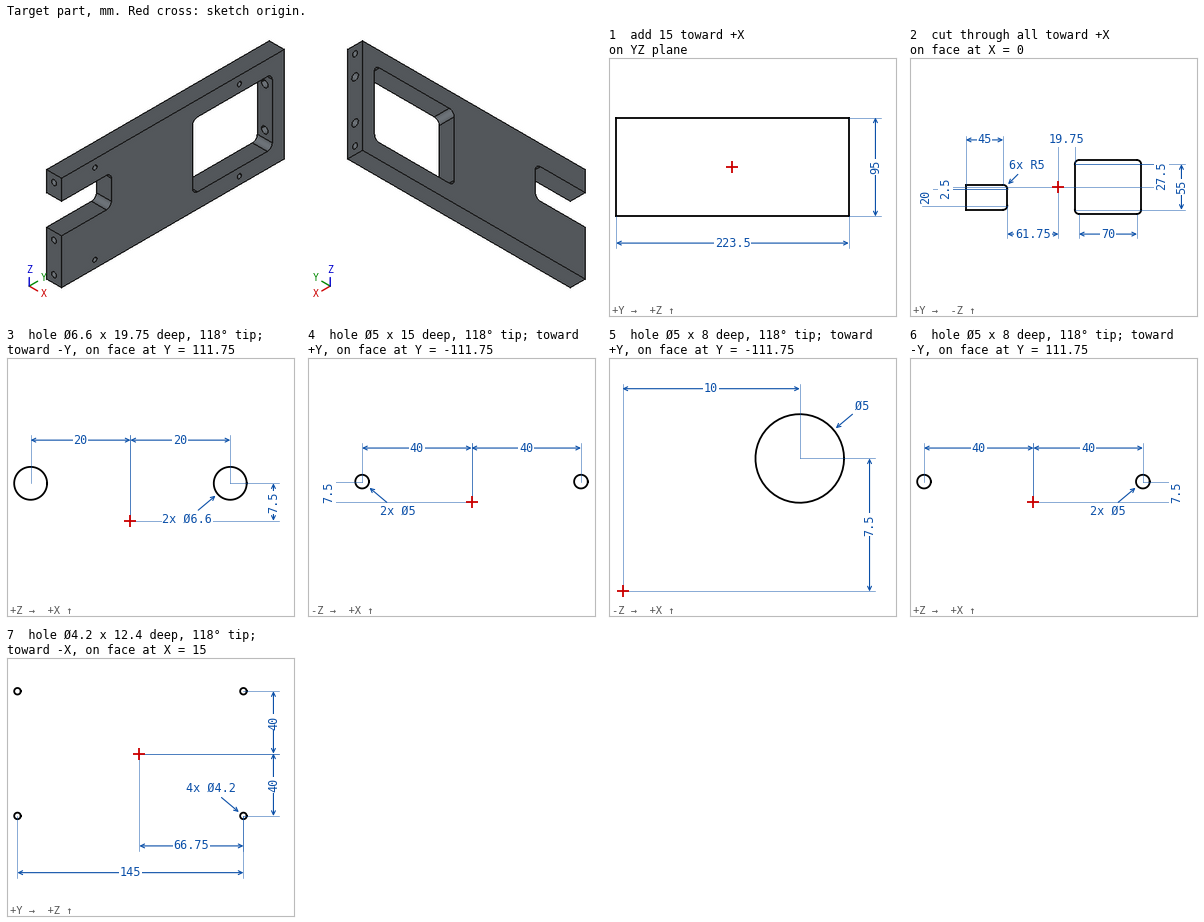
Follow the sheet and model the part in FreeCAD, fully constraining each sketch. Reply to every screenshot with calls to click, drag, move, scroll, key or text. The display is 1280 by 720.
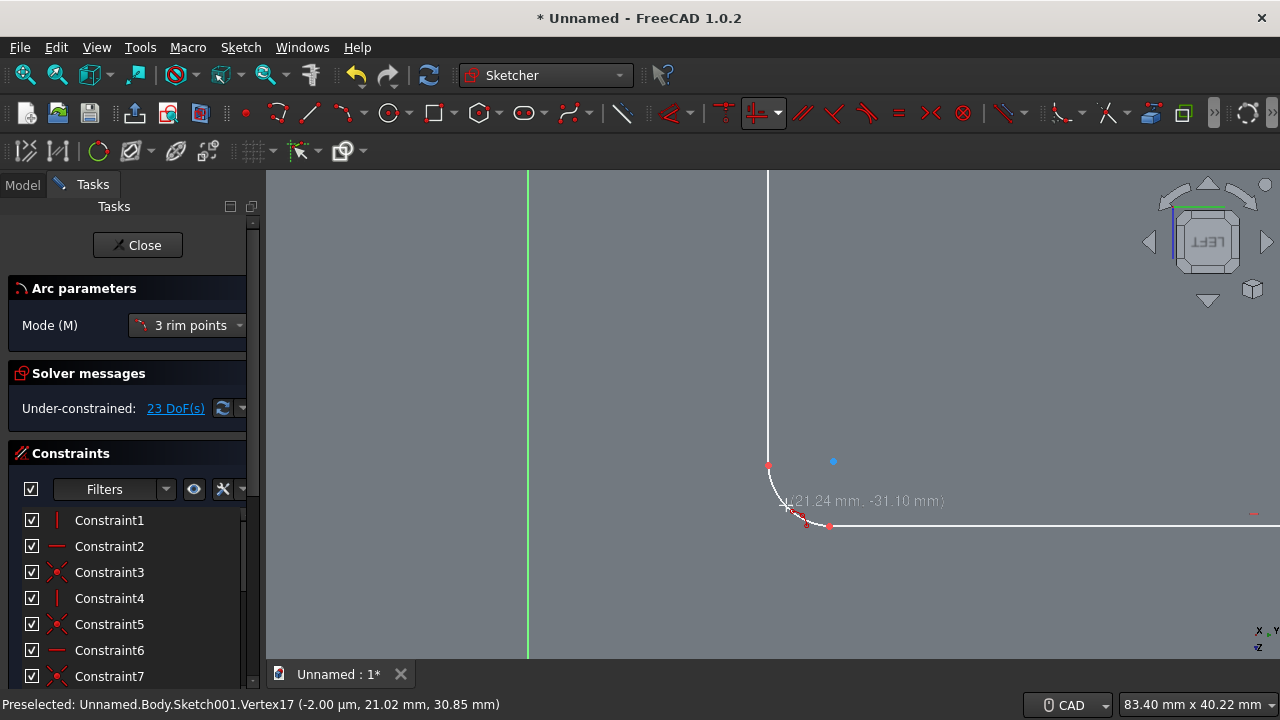
scroll(786, 508, down, 7)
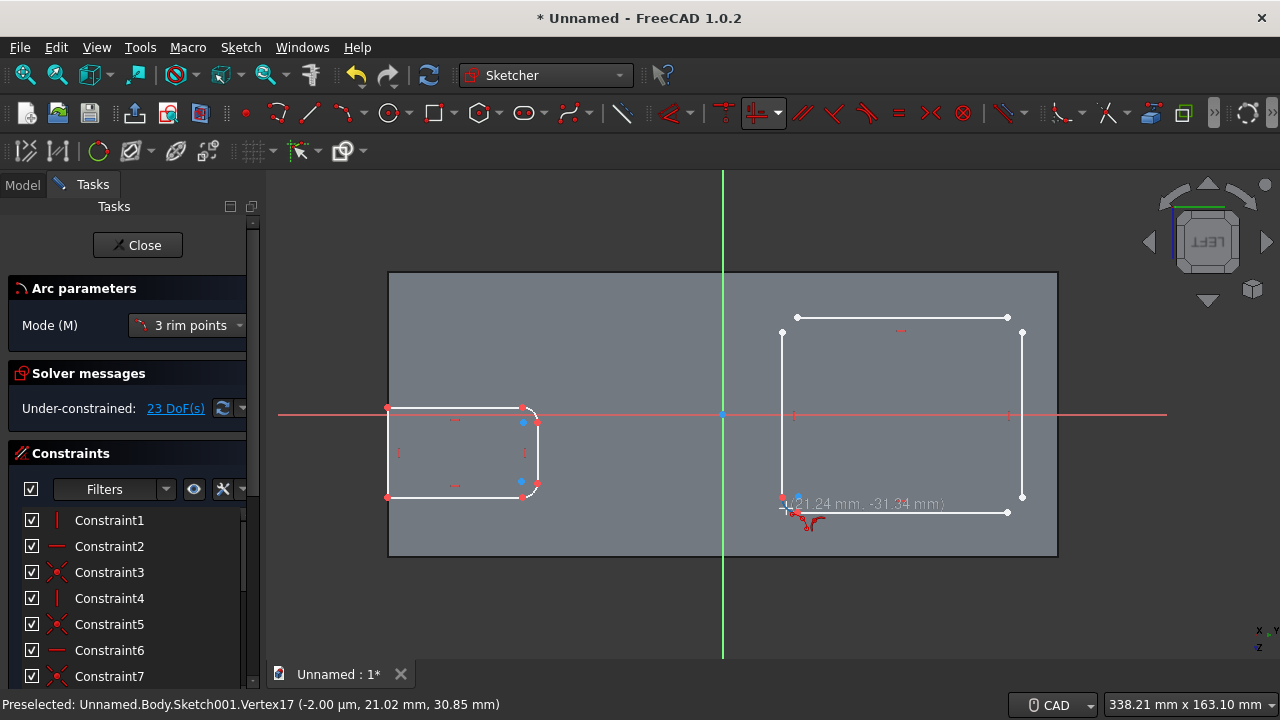
click(1007, 513)
click(1022, 498)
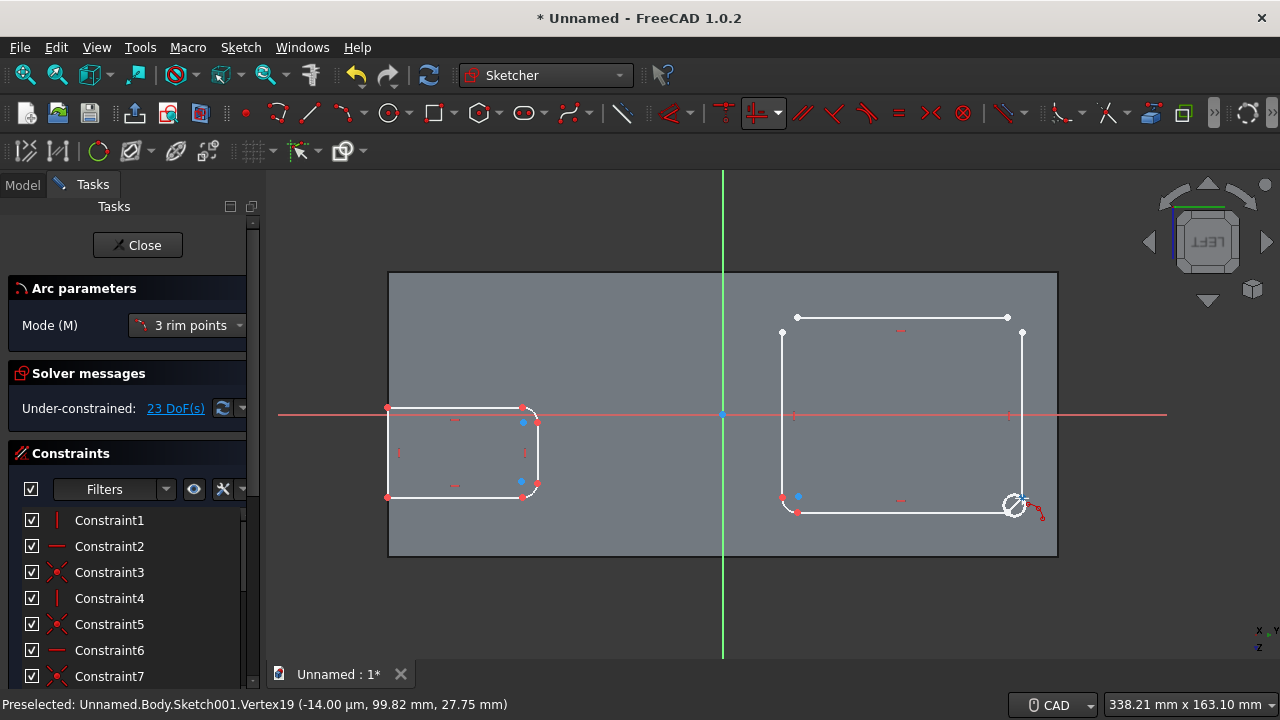
scroll(1017, 508, up, 7)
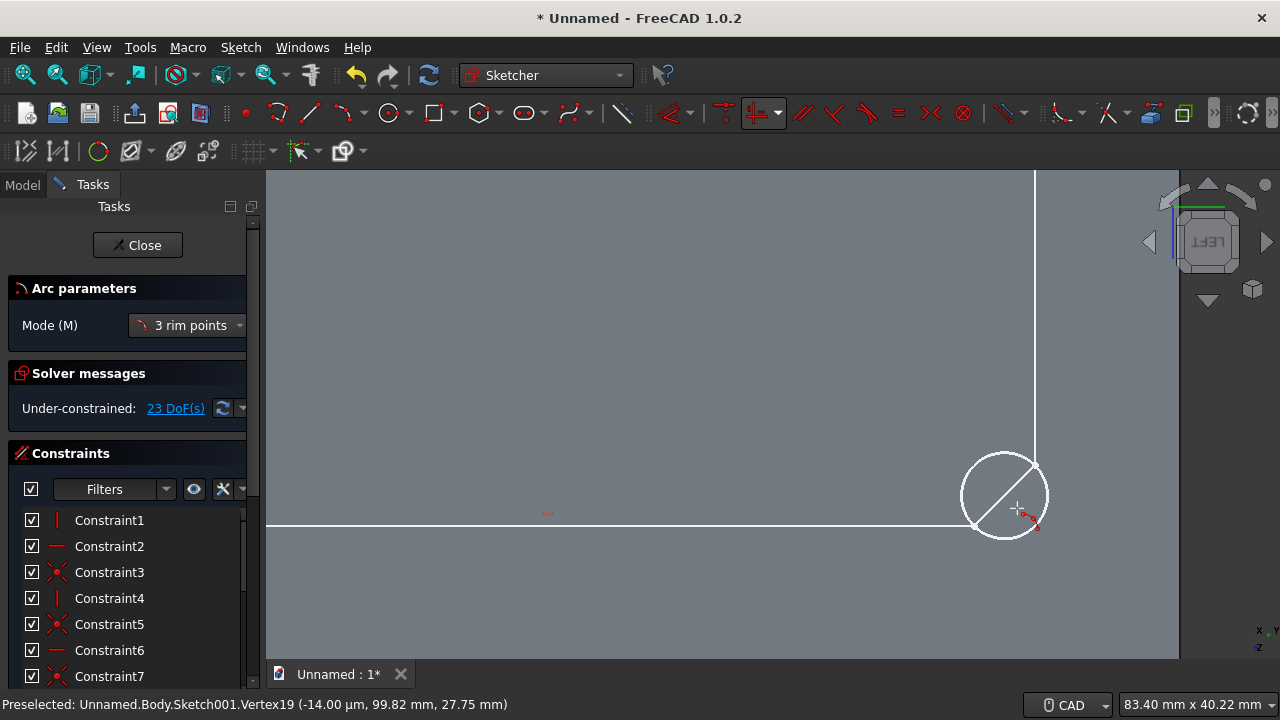
click(1016, 505)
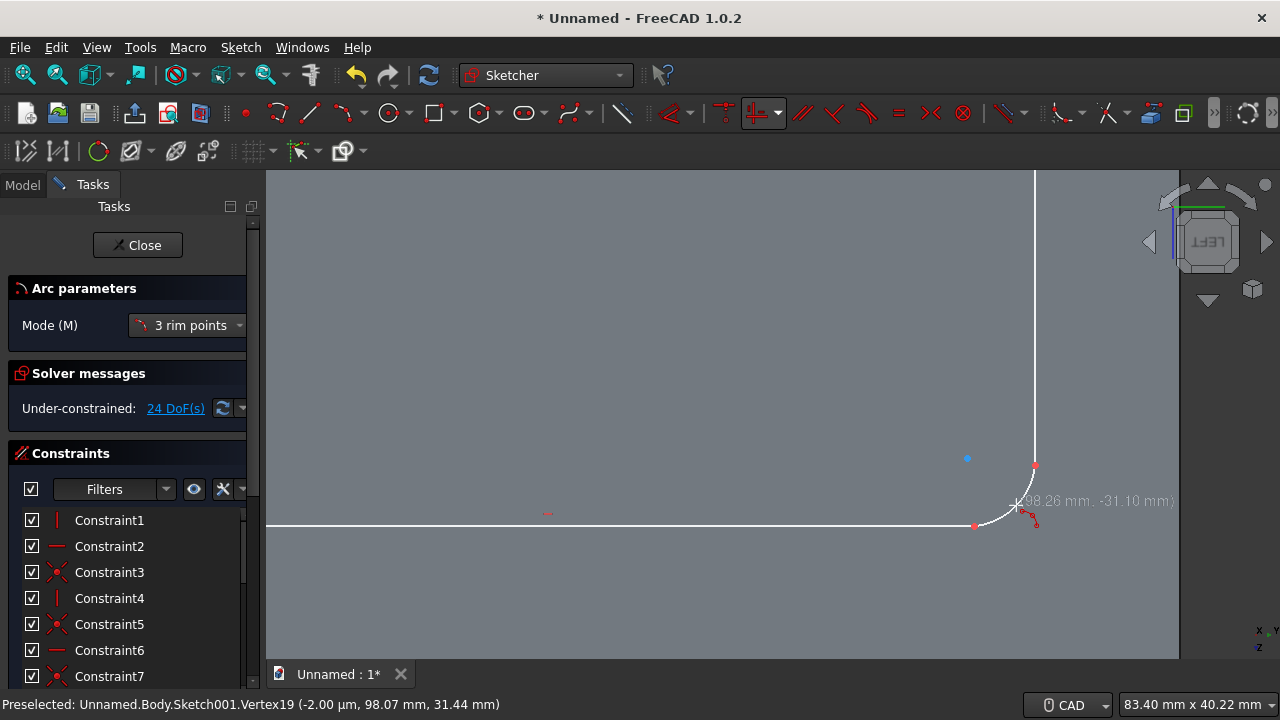
scroll(1017, 508, down, 7)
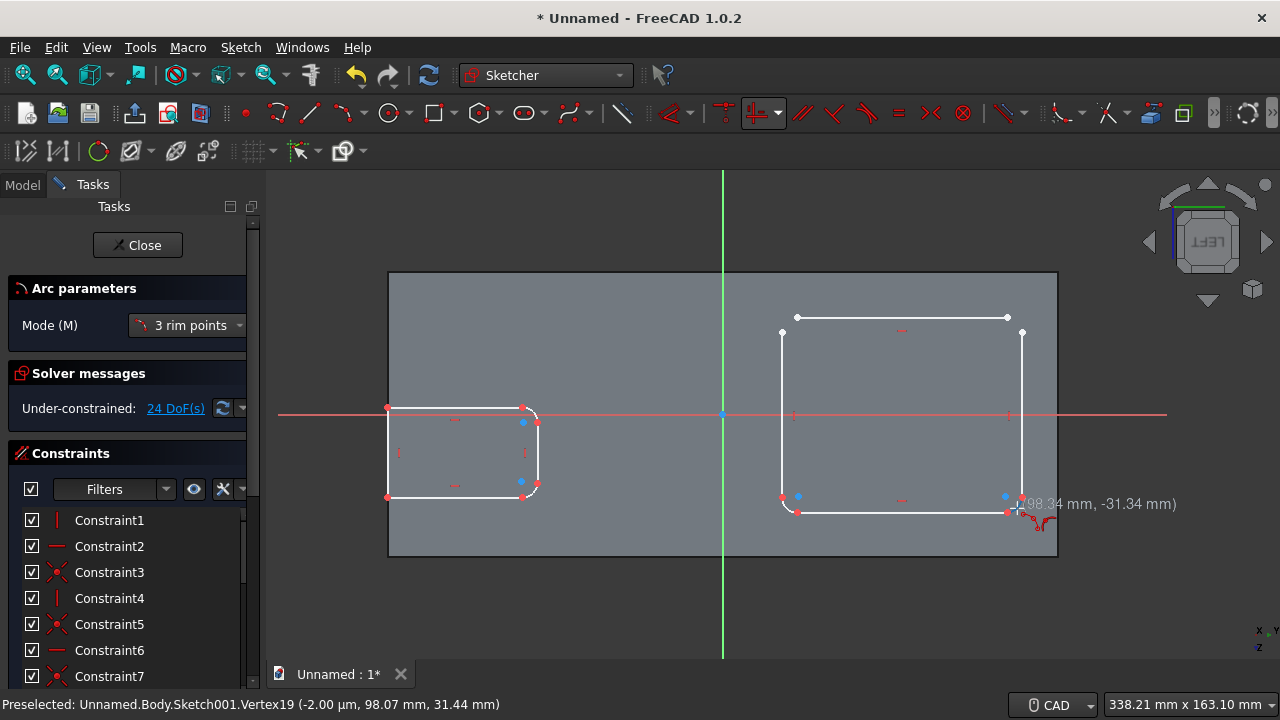
click(1022, 333)
click(1007, 318)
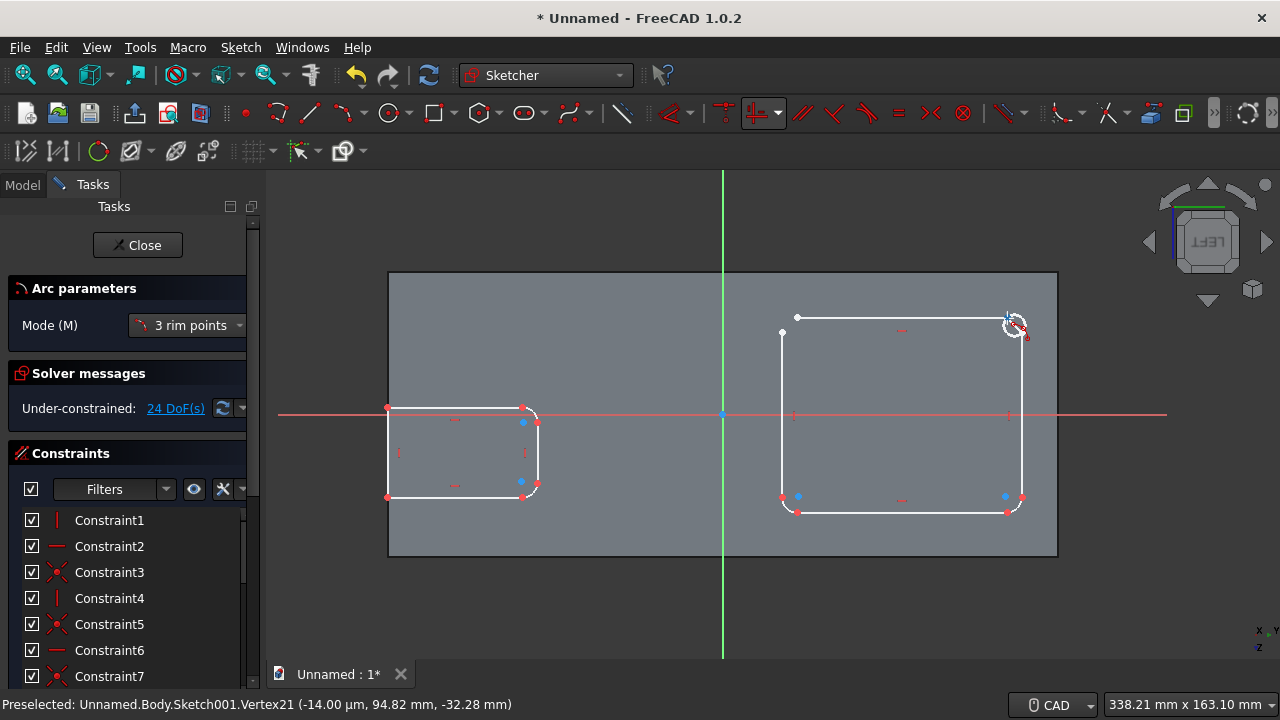
scroll(1017, 322, up, 7)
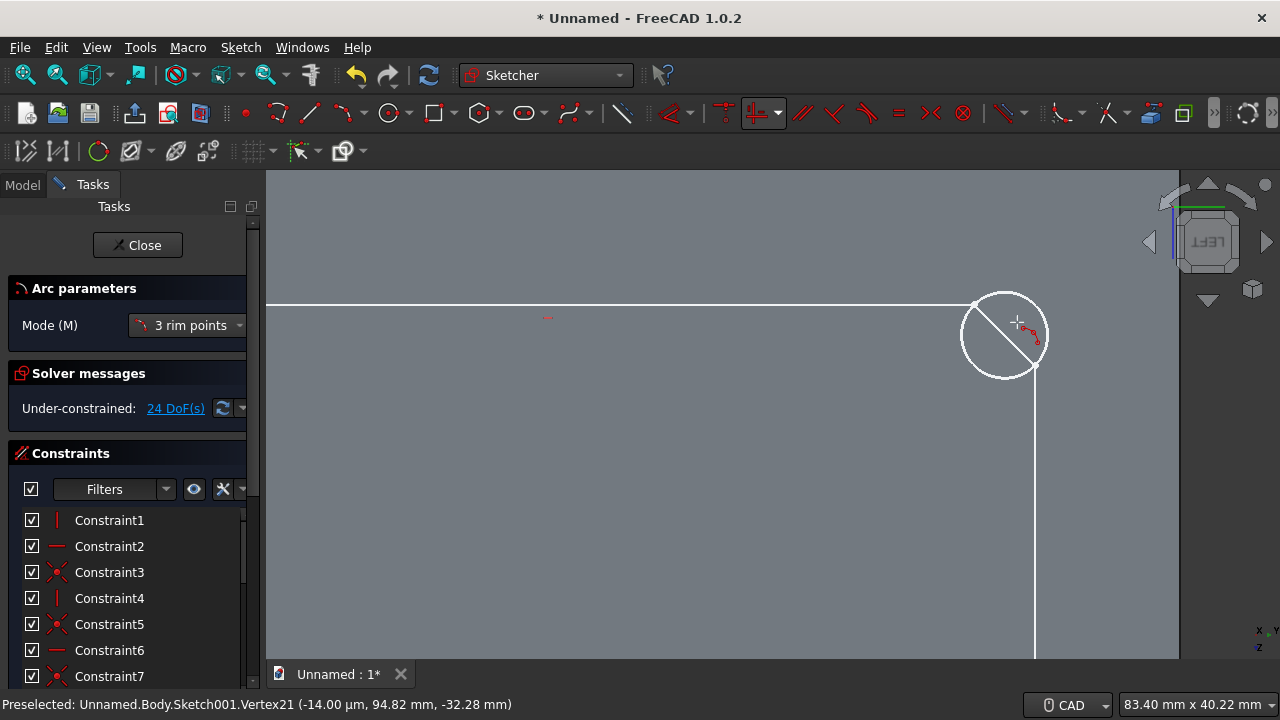
click(1016, 320)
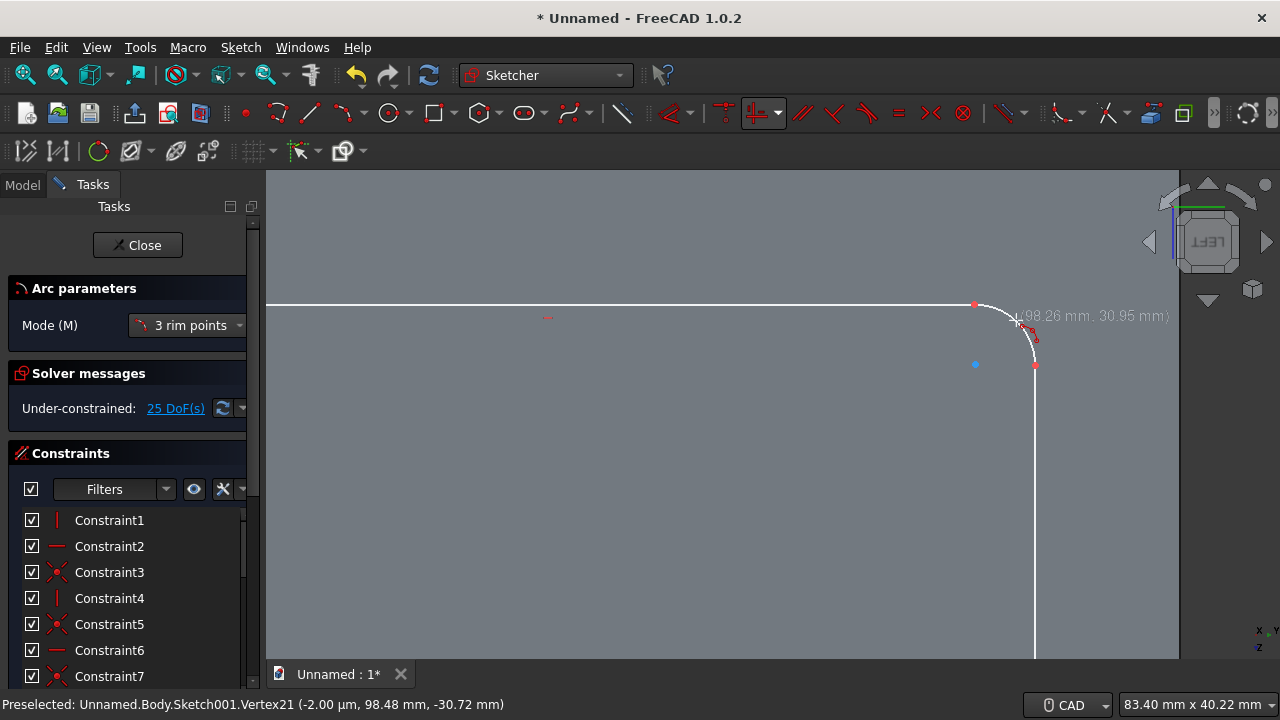
scroll(1017, 322, down, 7)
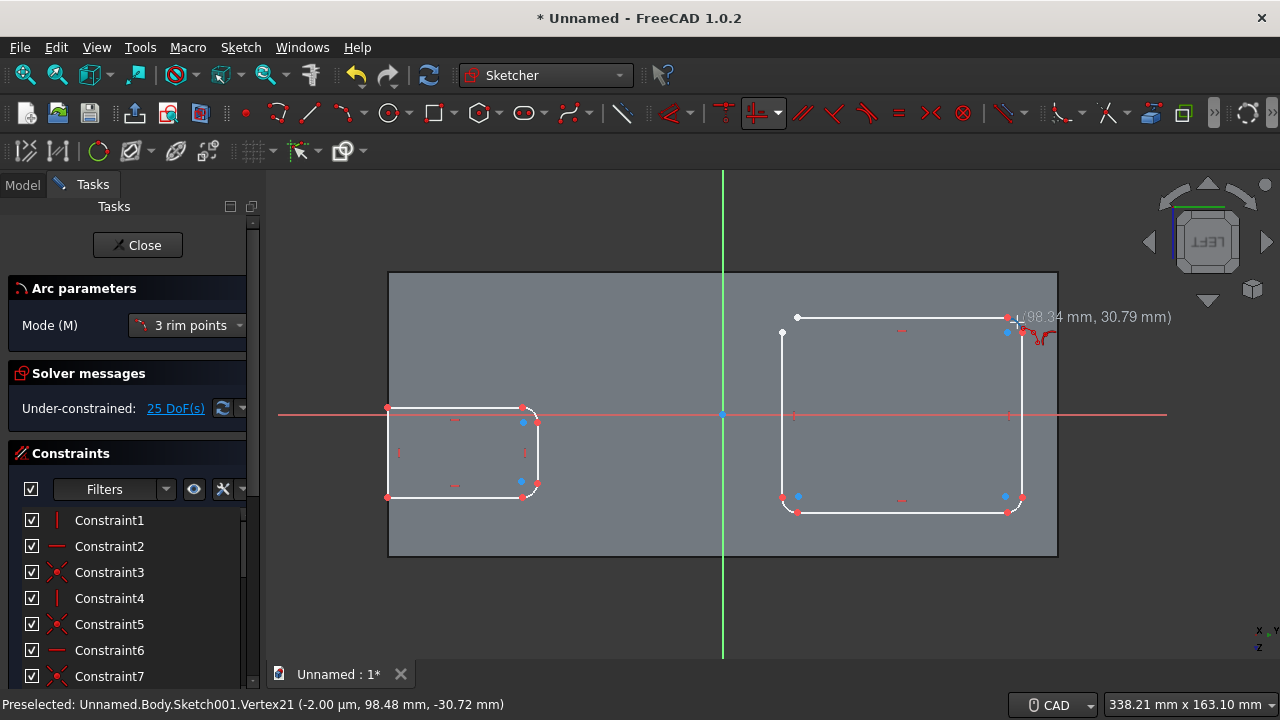
click(797, 318)
click(782, 333)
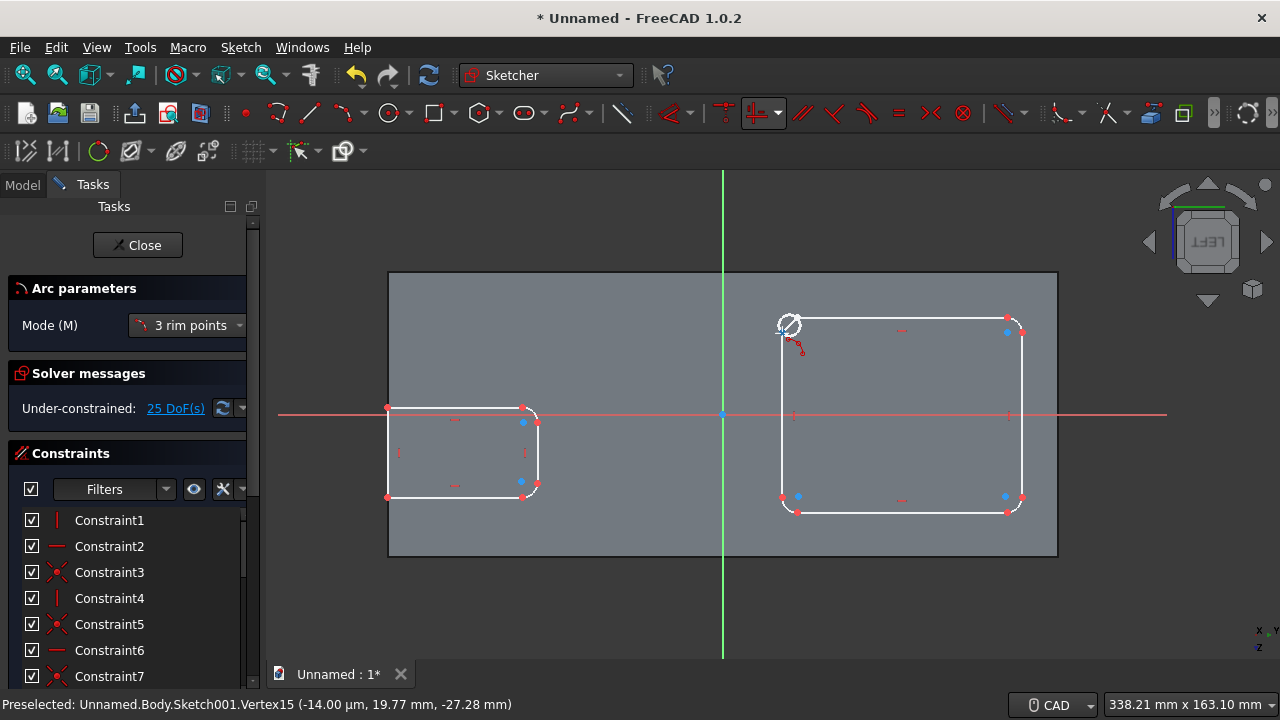
scroll(786, 322, up, 7)